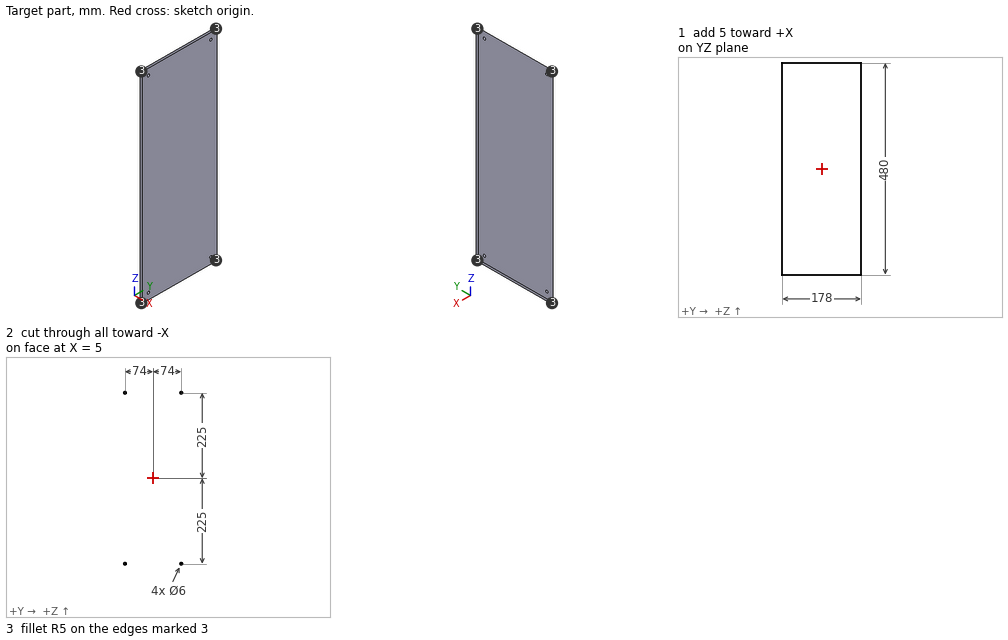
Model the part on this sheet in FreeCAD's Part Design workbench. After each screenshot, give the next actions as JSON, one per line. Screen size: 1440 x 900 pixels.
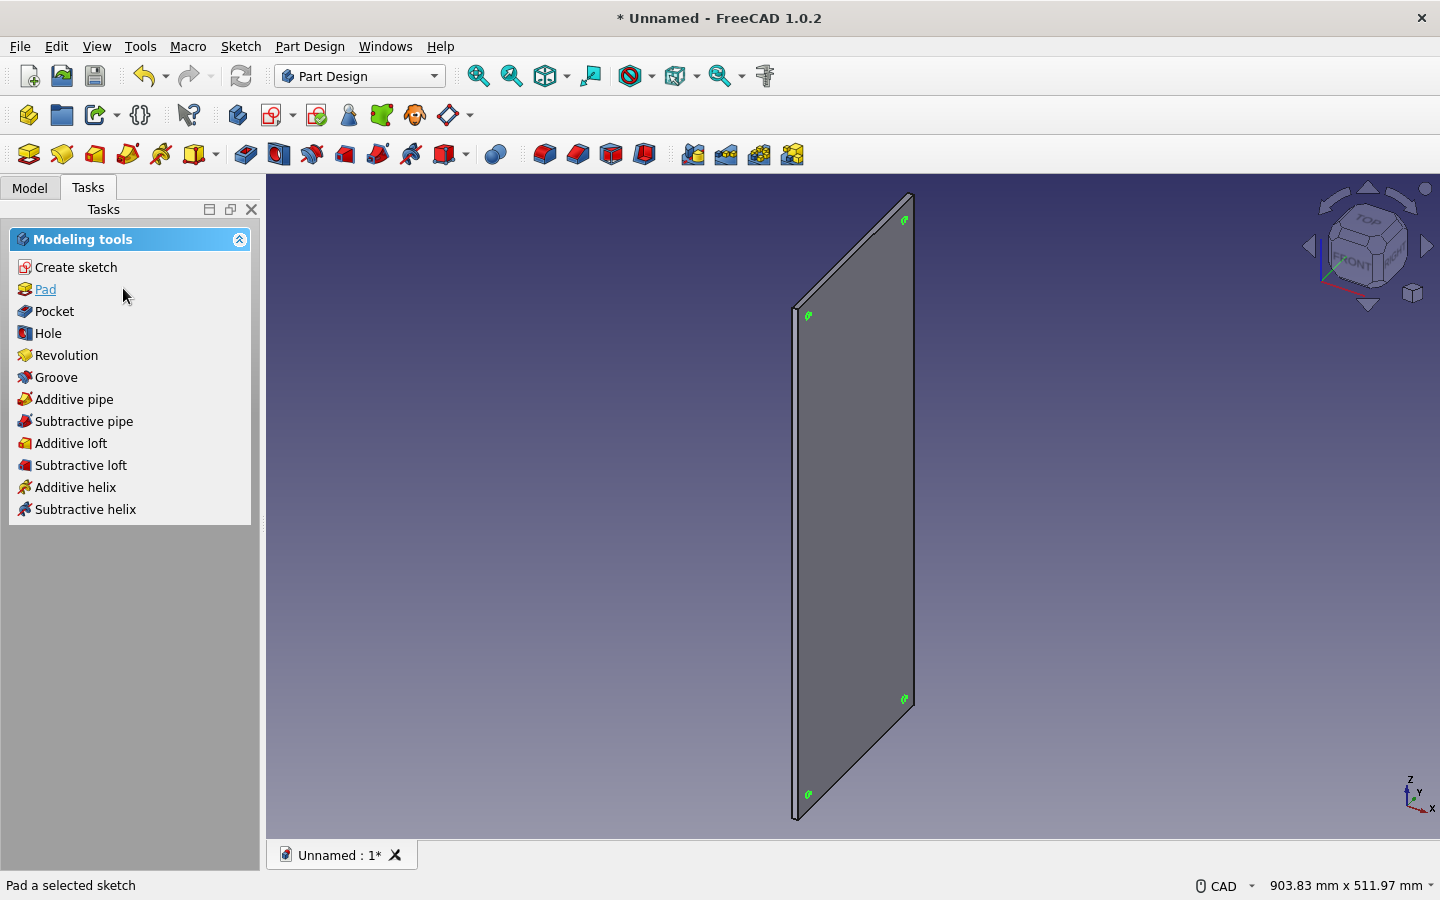
{"action": "left_click", "coordinate": [246, 154]}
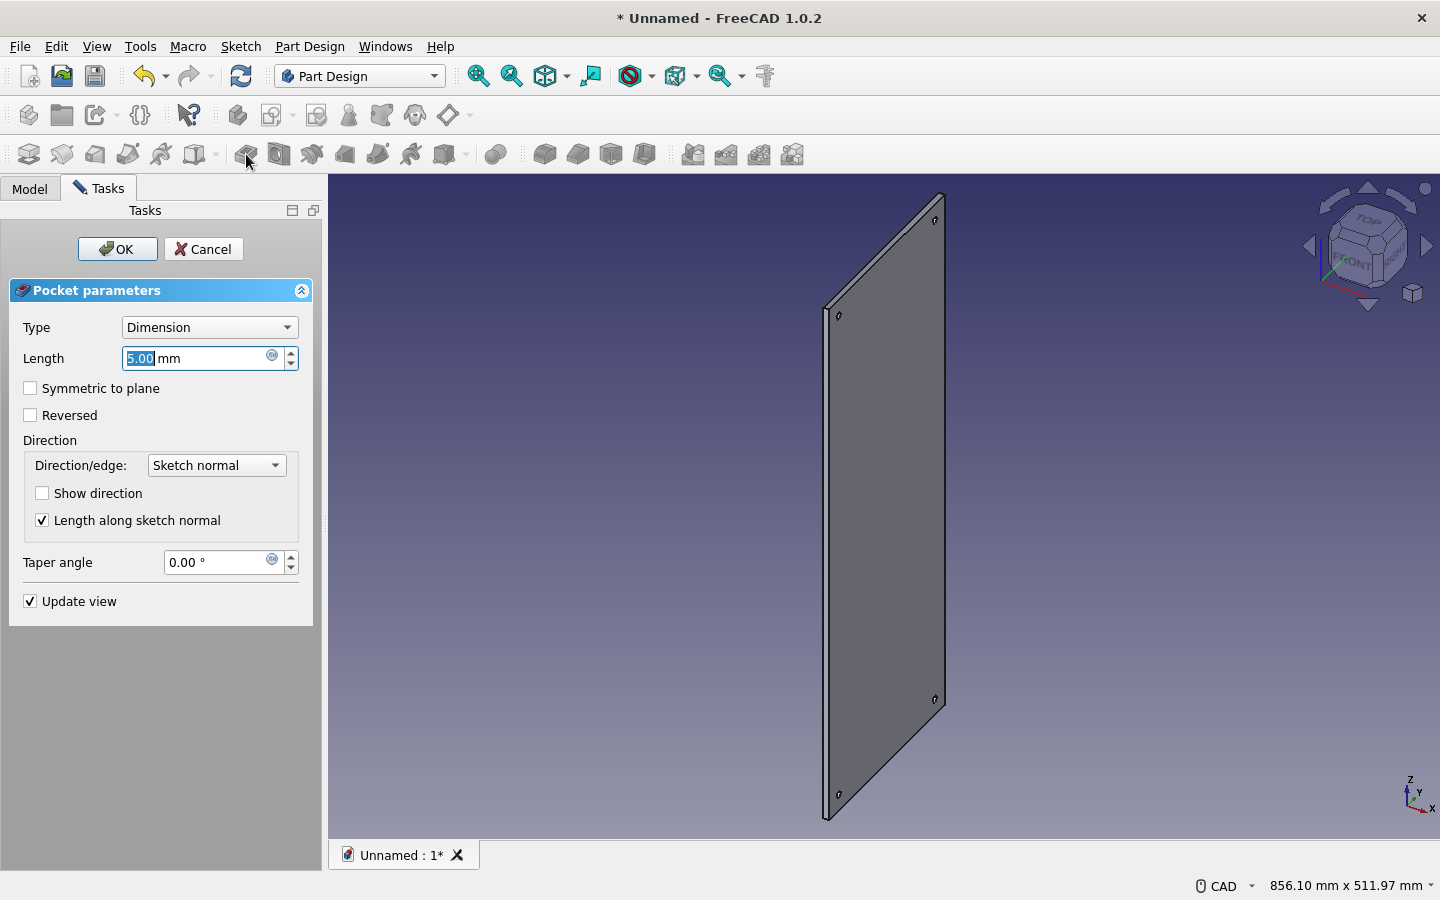
{"action": "left_click", "coordinate": [210, 328]}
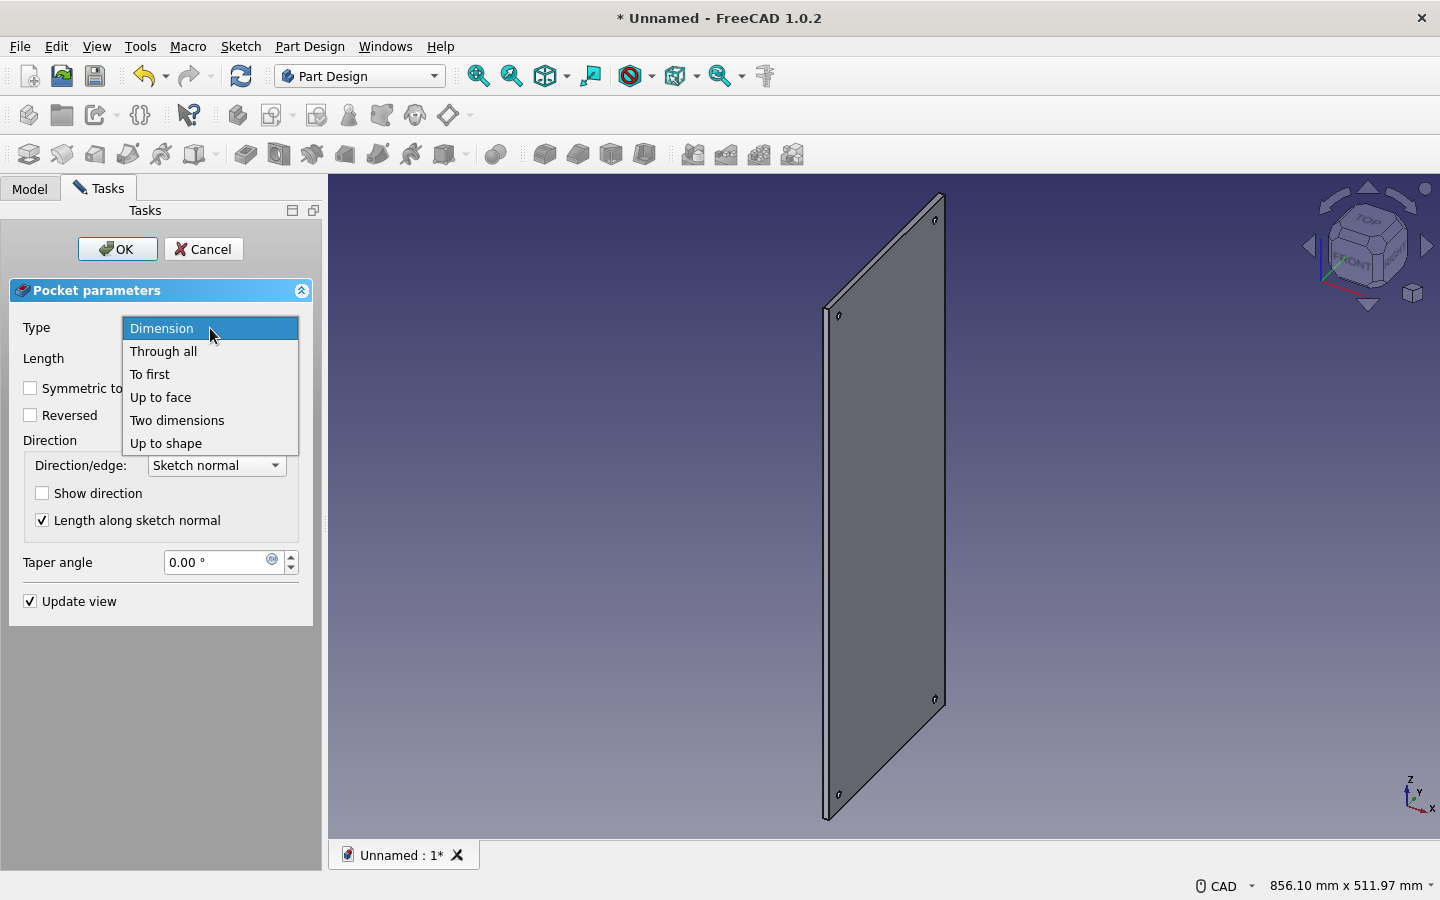
{"action": "left_click", "coordinate": [208, 352]}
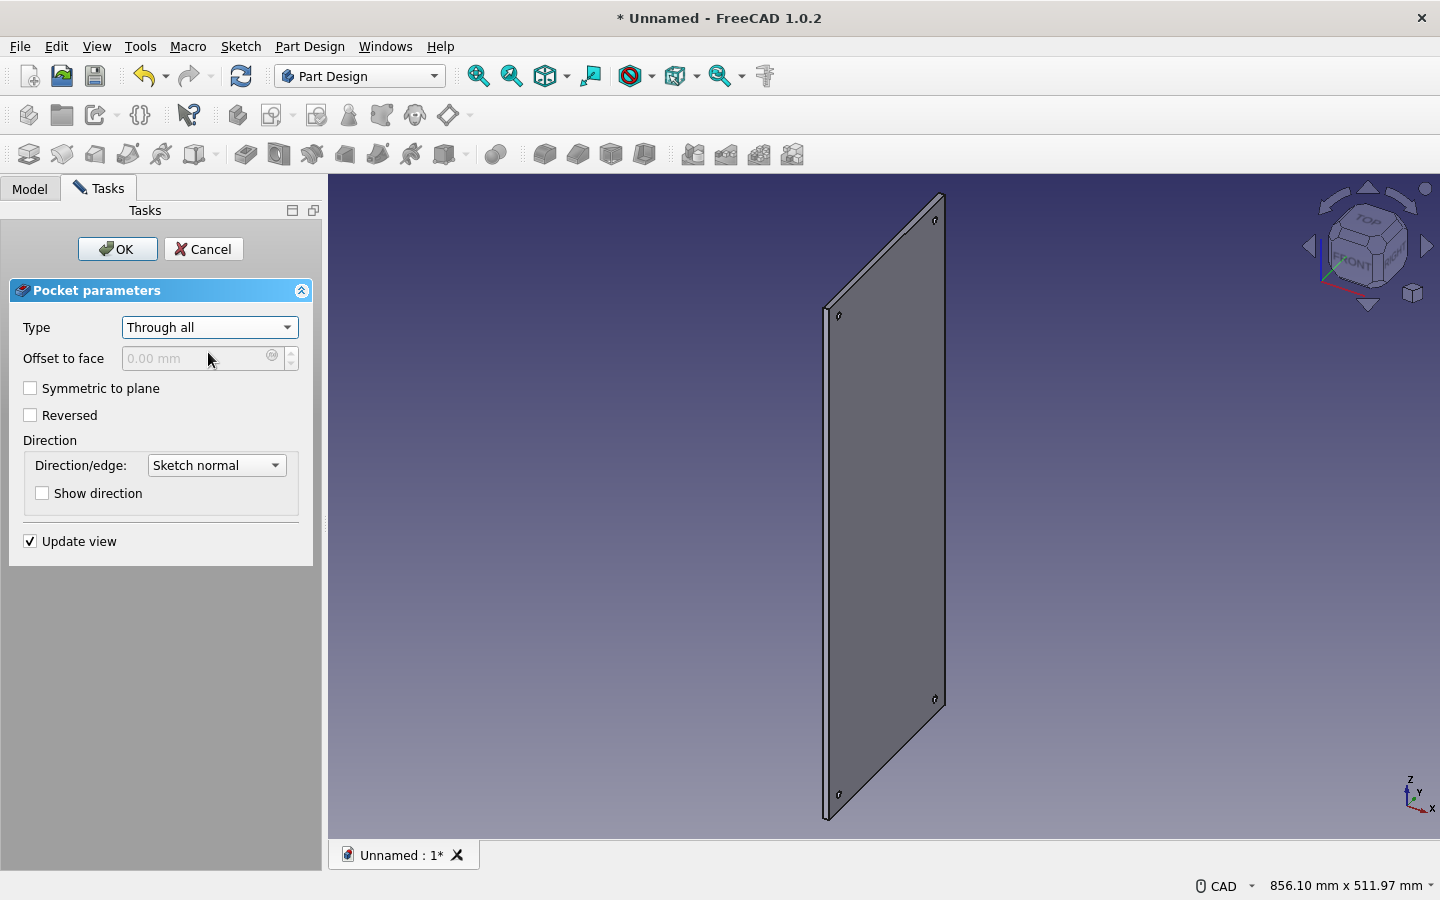
{"action": "left_click", "coordinate": [118, 249]}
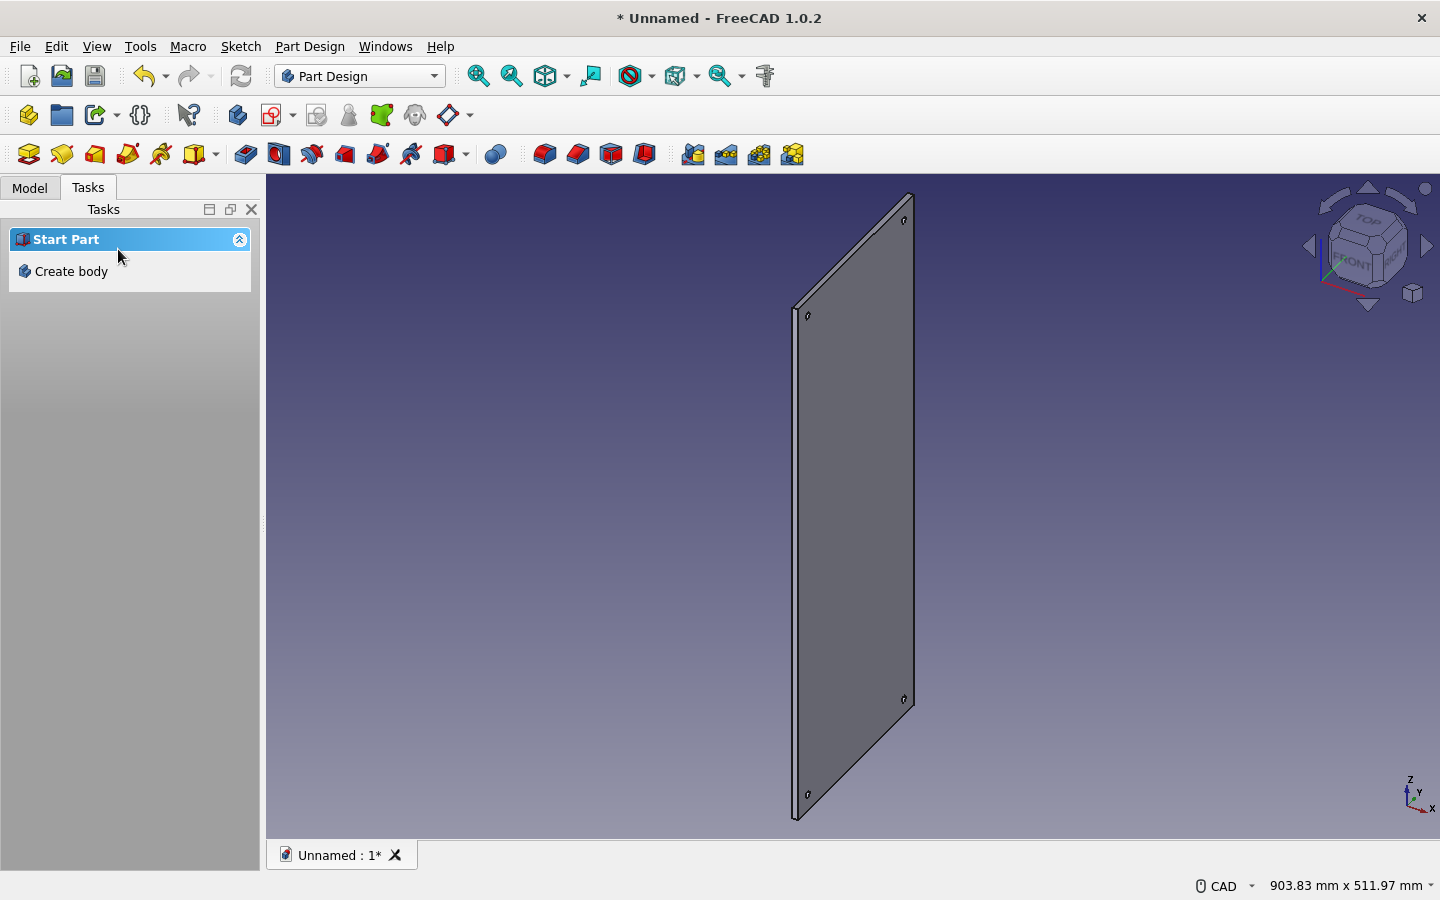
{"action": "key", "text": "0"}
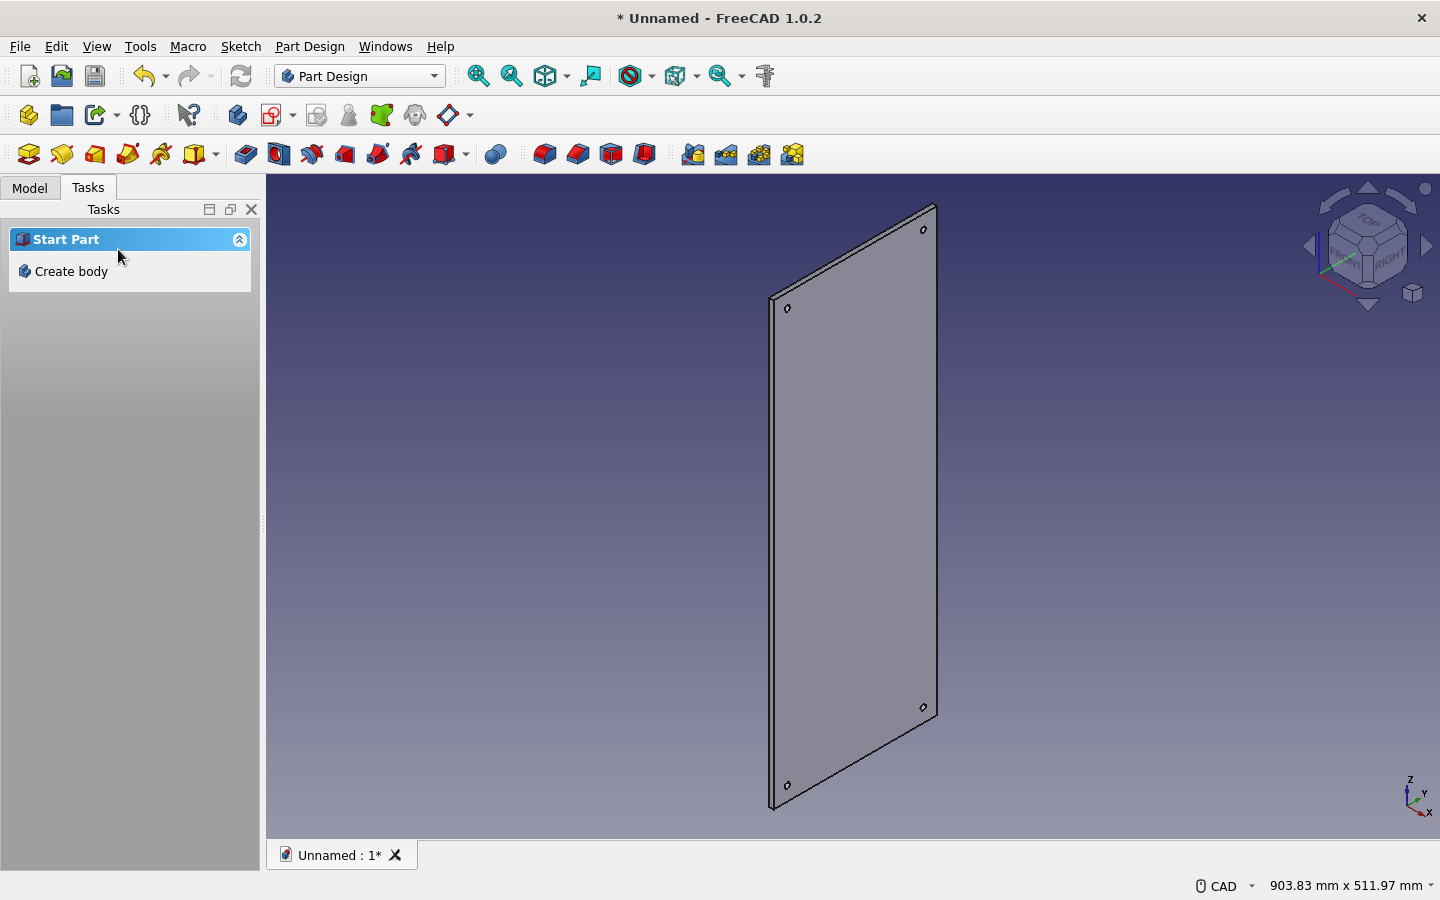
{"action": "scroll", "coordinate": [935, 204], "scroll_direction": "up", "scroll_amount": 10}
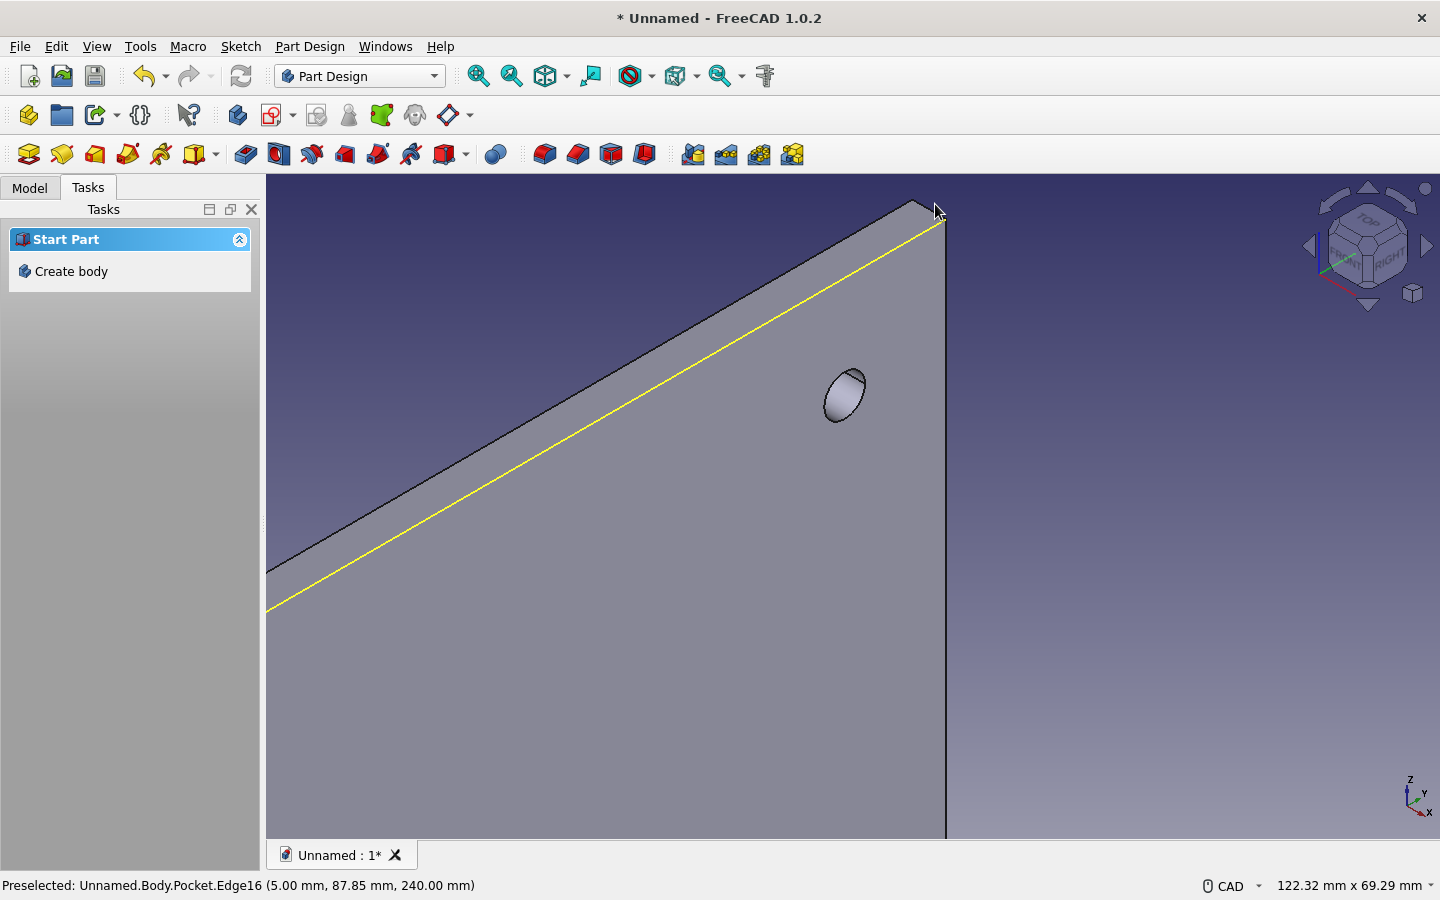
{"action": "left_click", "coordinate": [479, 76]}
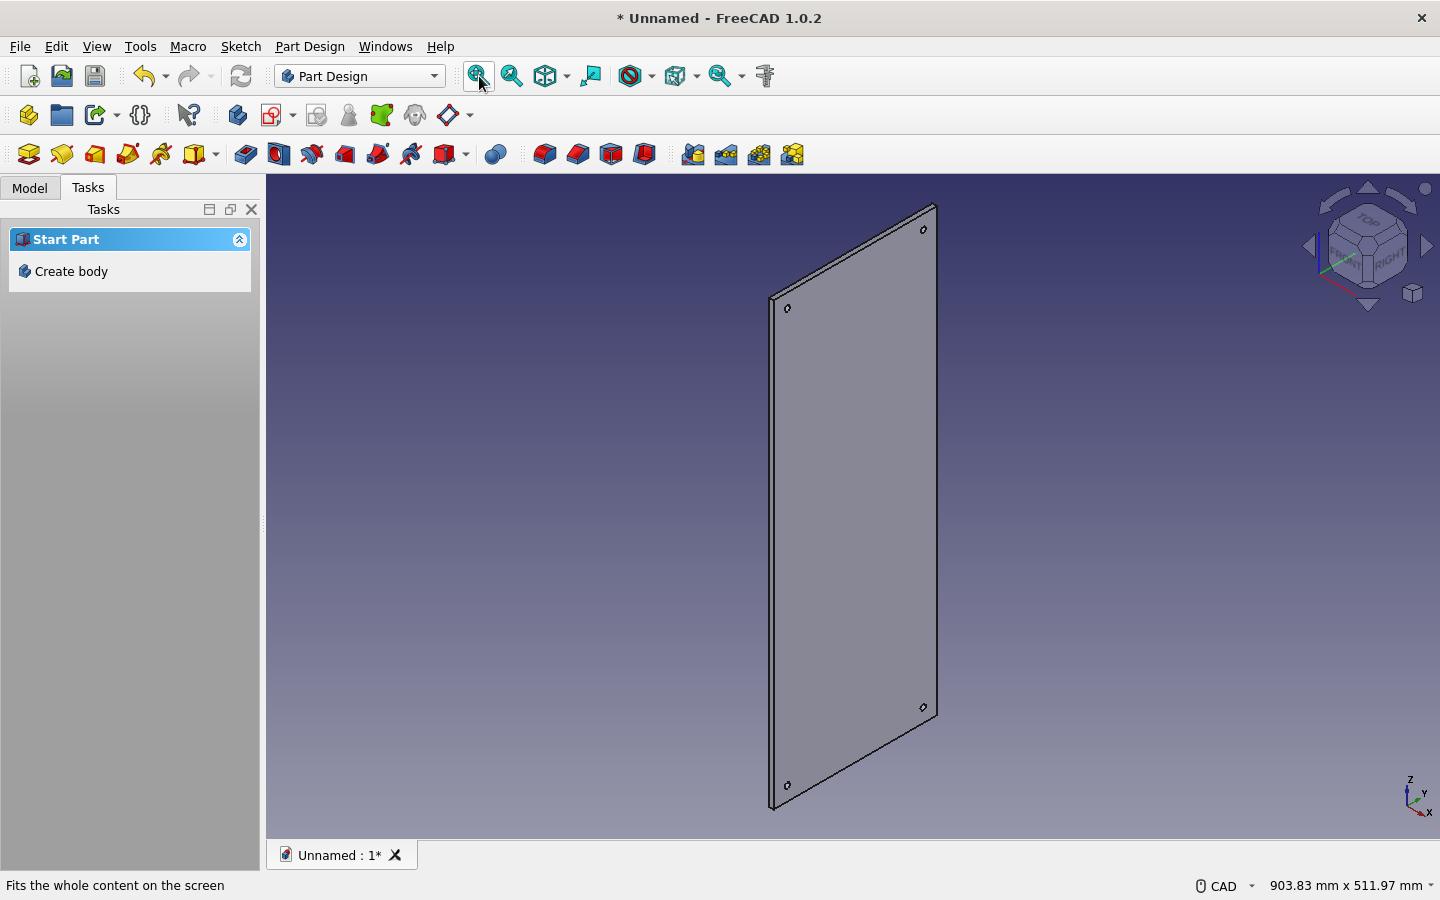
{"action": "key", "text": "2"}